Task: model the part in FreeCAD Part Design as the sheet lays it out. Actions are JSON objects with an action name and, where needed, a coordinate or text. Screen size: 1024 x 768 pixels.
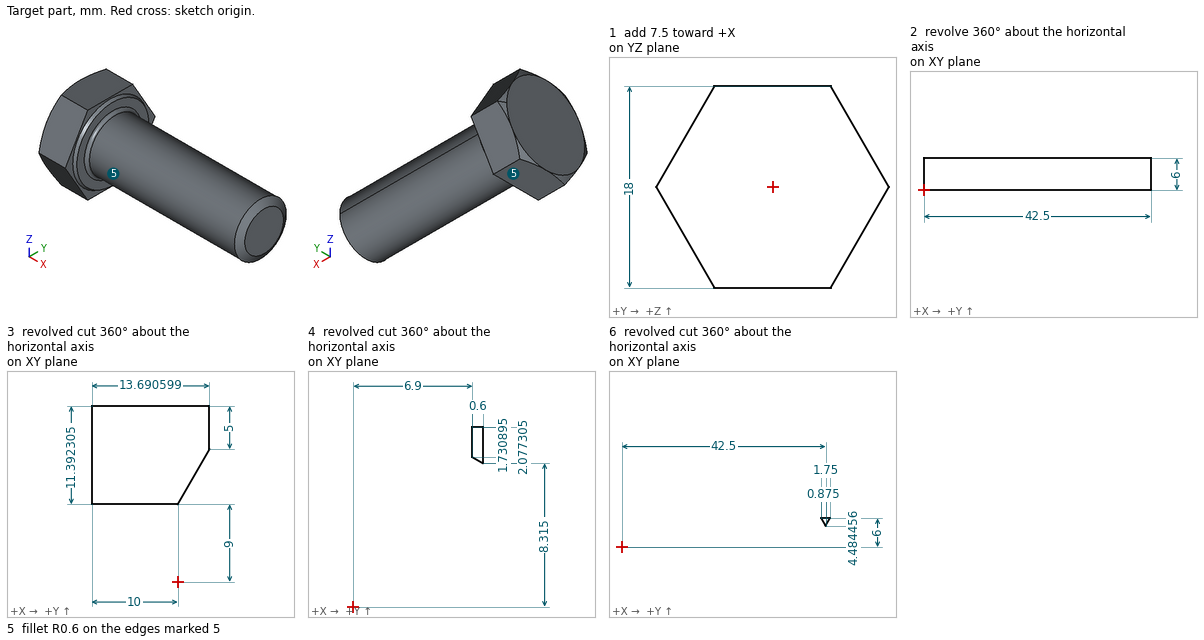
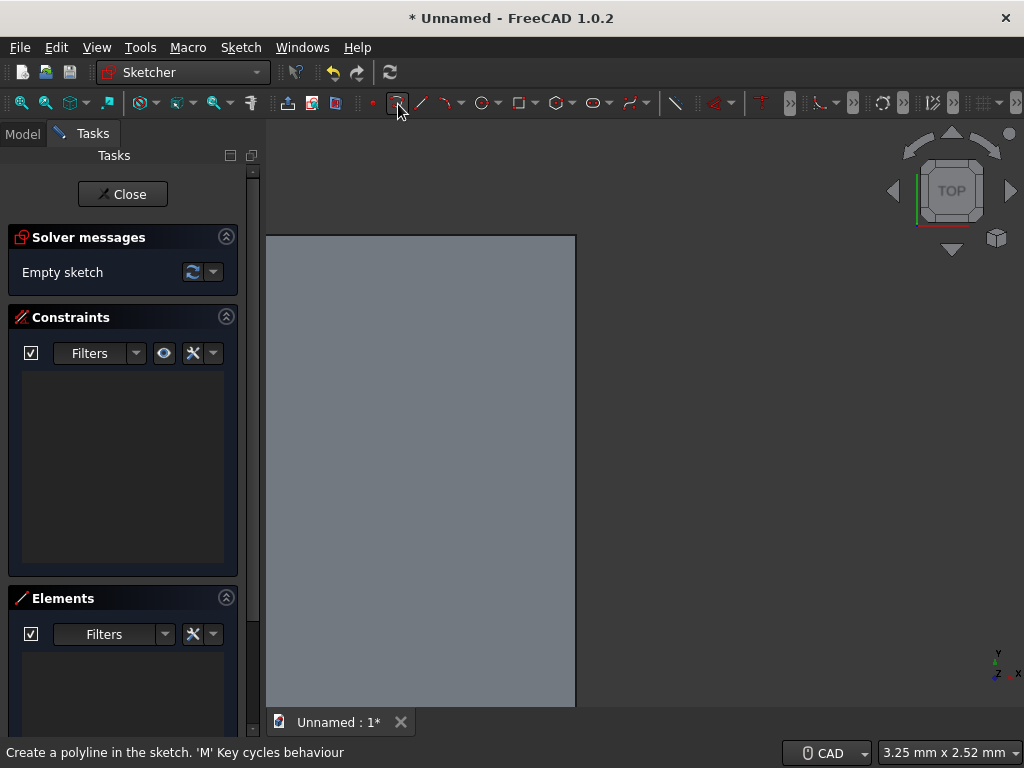
{"action": "left_click", "coordinate": [372, 235]}
{"action": "left_click", "coordinate": [576, 589]}
{"action": "left_click", "coordinate": [780, 235]}
{"action": "left_click", "coordinate": [372, 236]}
{"action": "key", "text": "Escape"}
{"action": "key", "text": "Escape"}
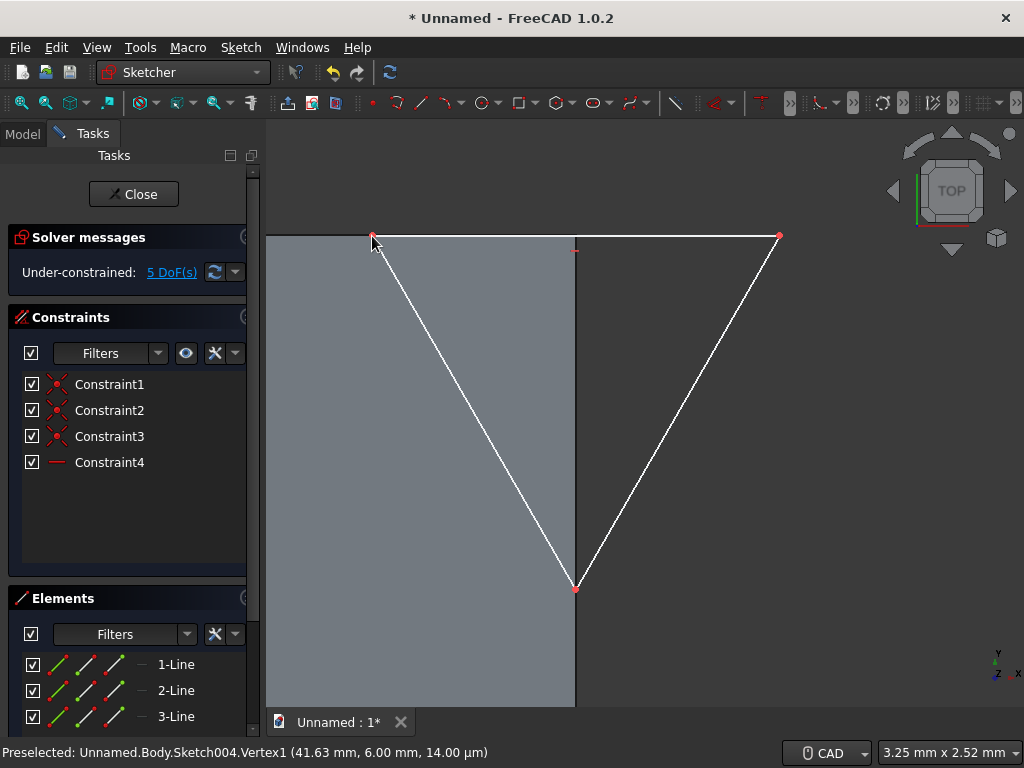
{"action": "left_click", "coordinate": [714, 104]}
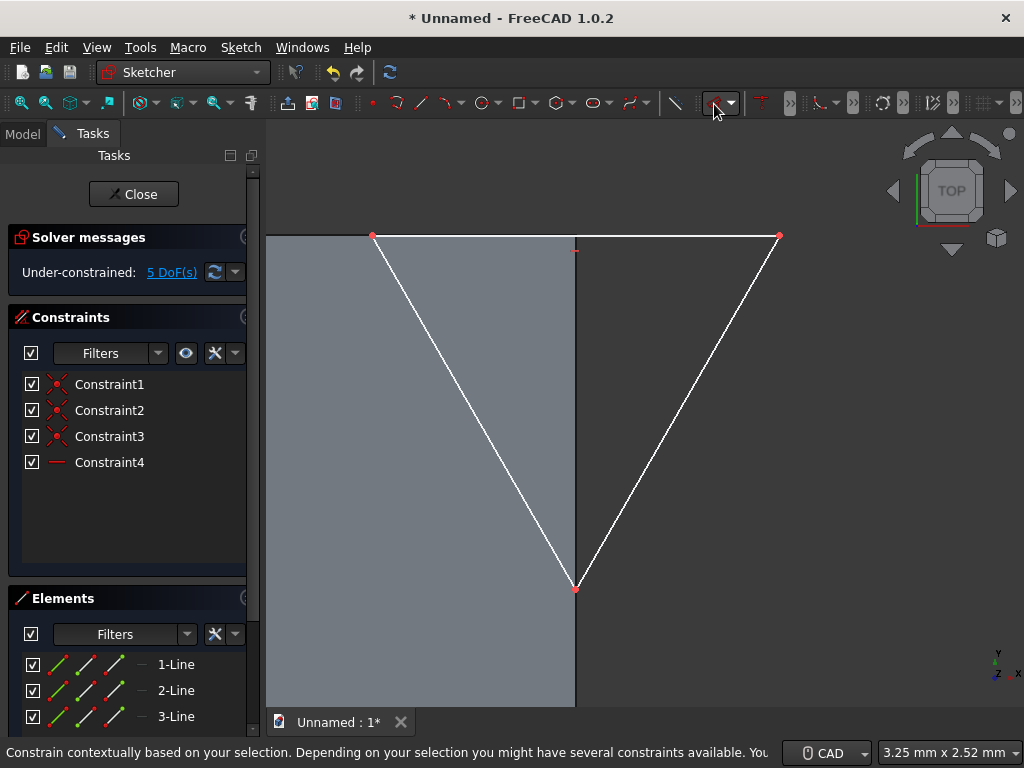
{"action": "left_click", "coordinate": [372, 236]}
{"action": "left_click", "coordinate": [406, 458]}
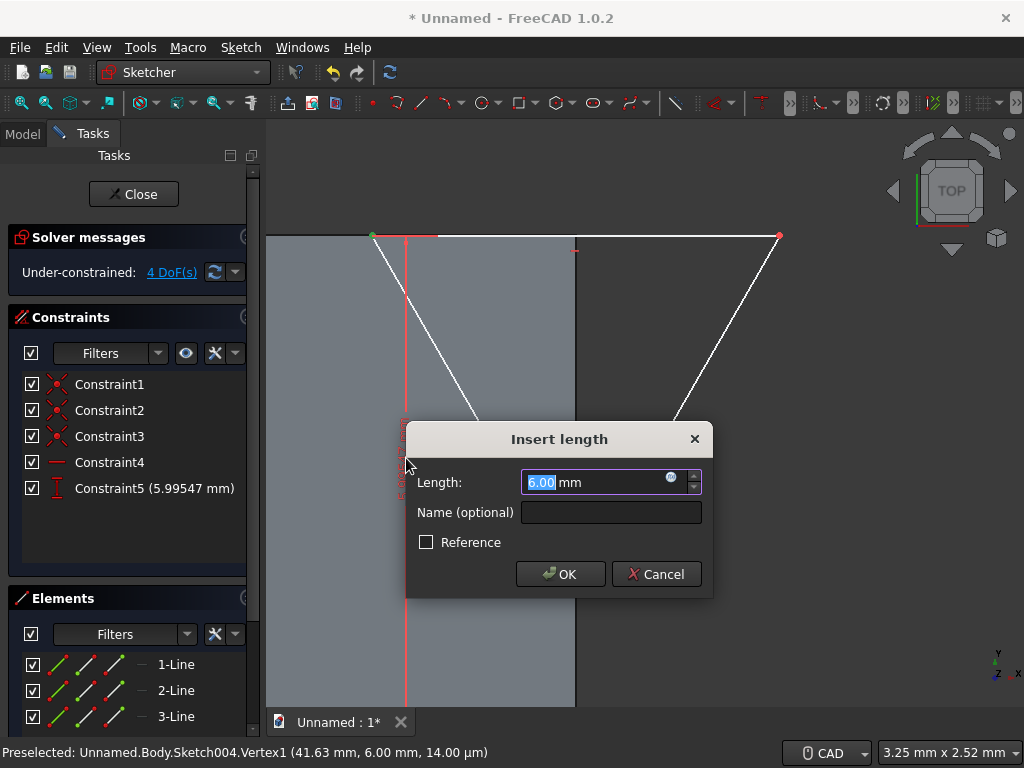
{"action": "type", "text": "6"}
{"action": "key", "text": "Return"}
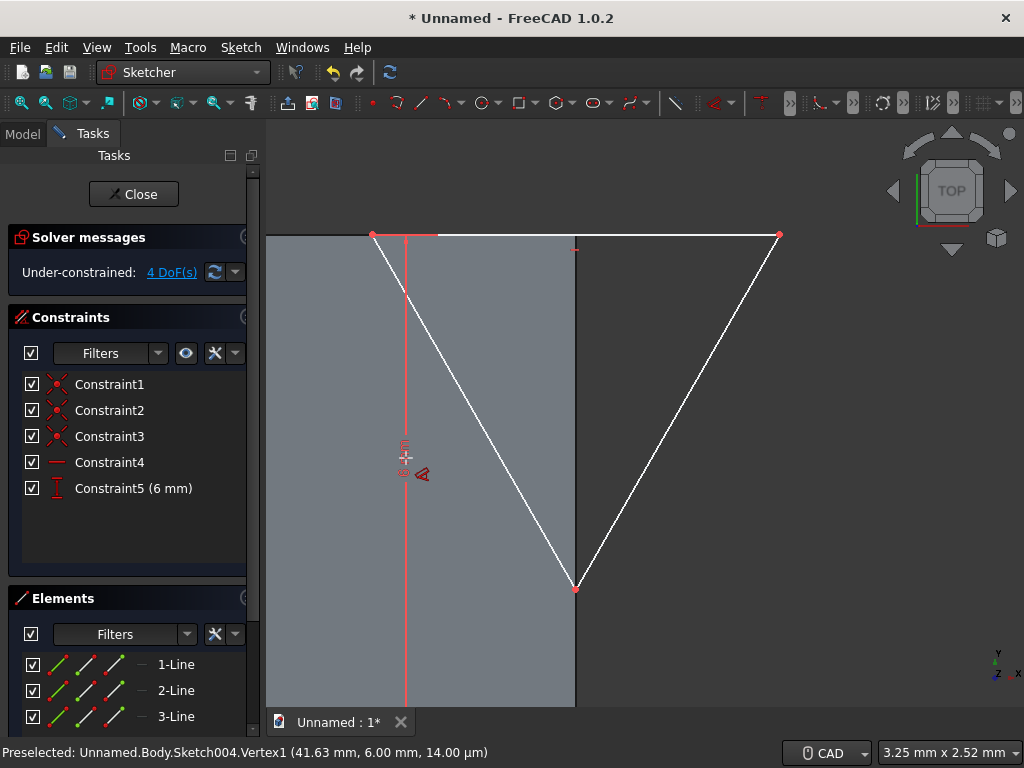
{"action": "left_click", "coordinate": [658, 235]}
{"action": "left_click", "coordinate": [576, 201]}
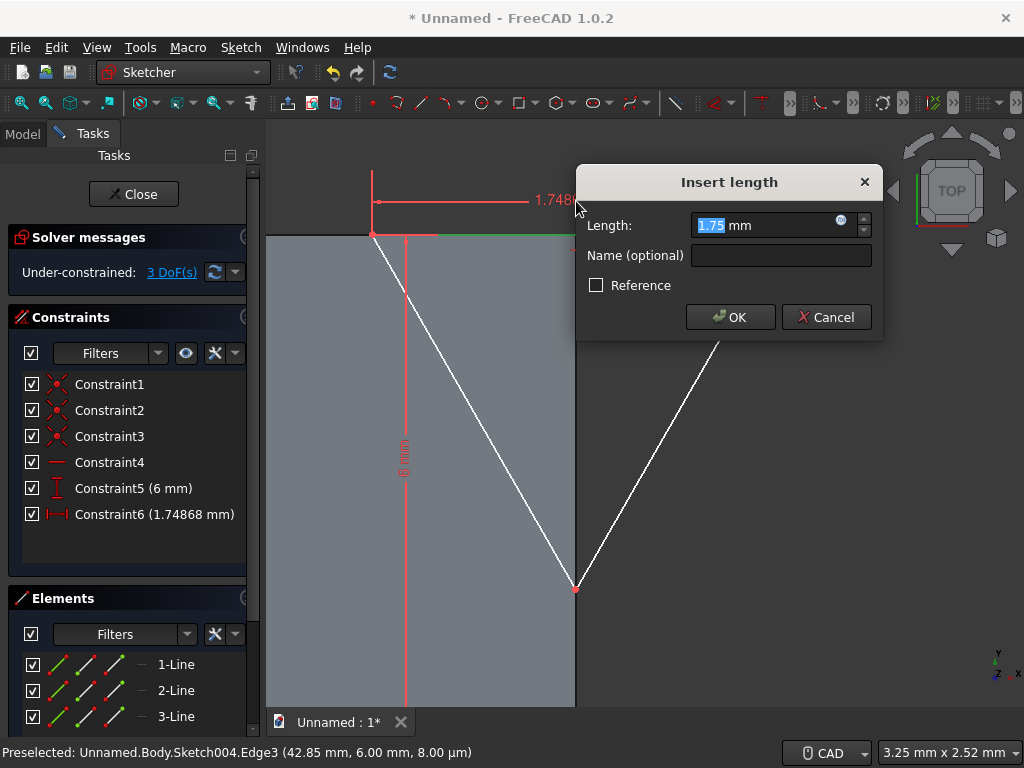
{"action": "type", "text": "1.75"}
{"action": "key", "text": "Return"}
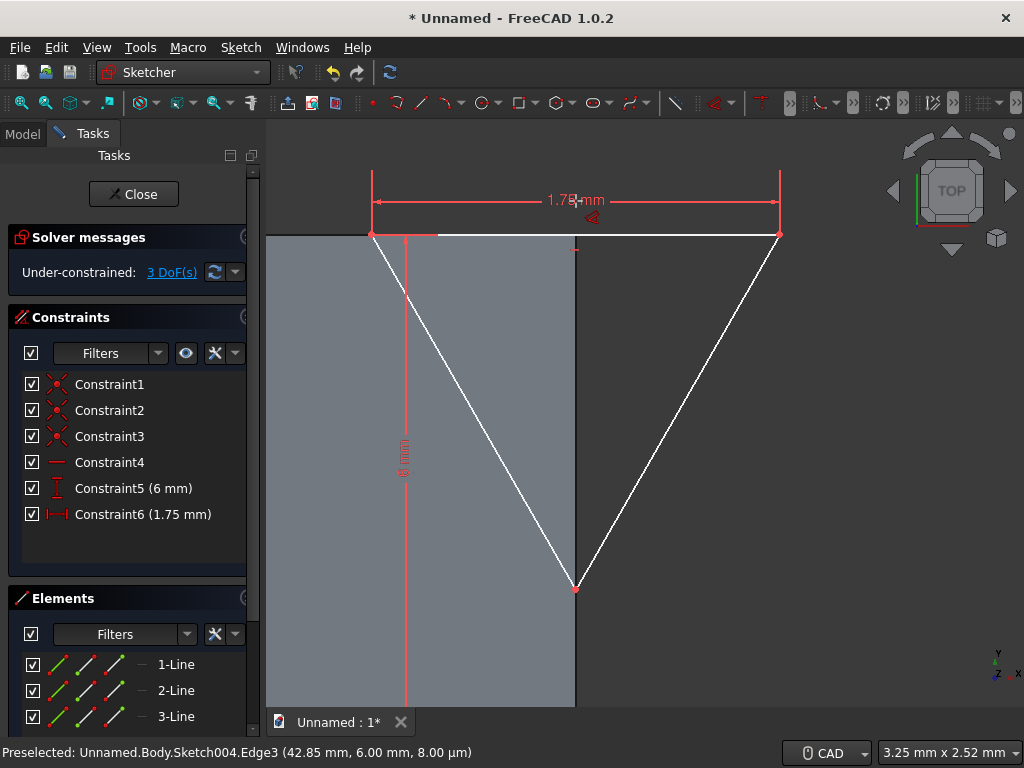
{"action": "left_click", "coordinate": [576, 590]}
{"action": "left_click", "coordinate": [435, 556]}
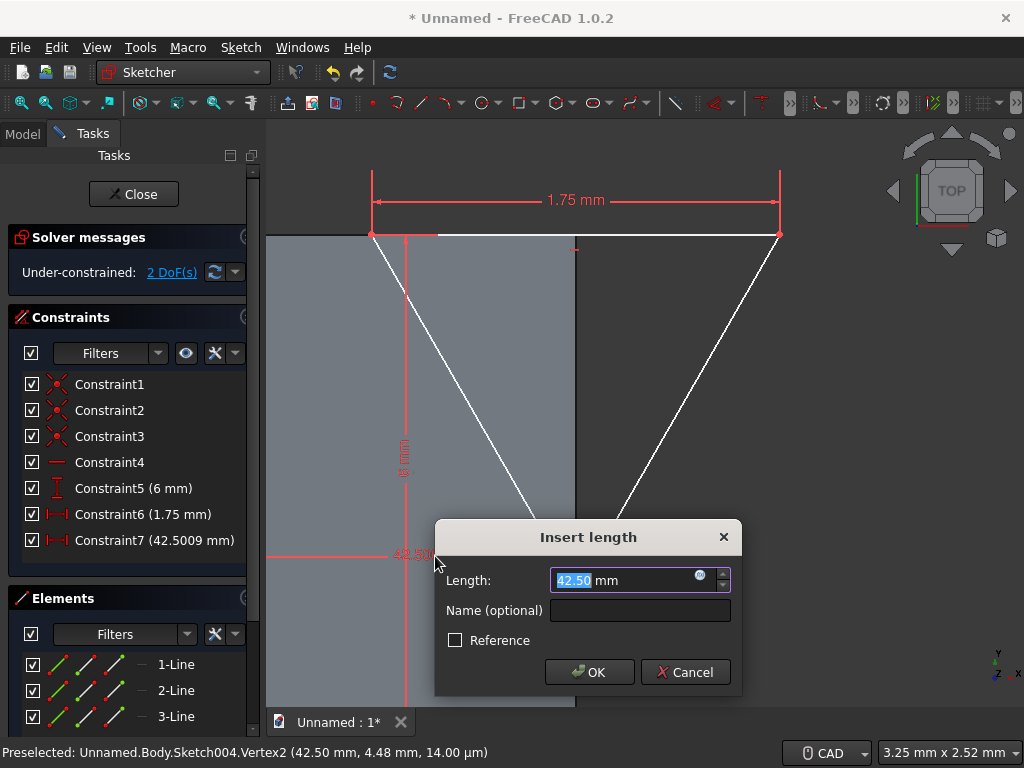
{"action": "type", "text": "42.5"}
{"action": "key", "text": "Return"}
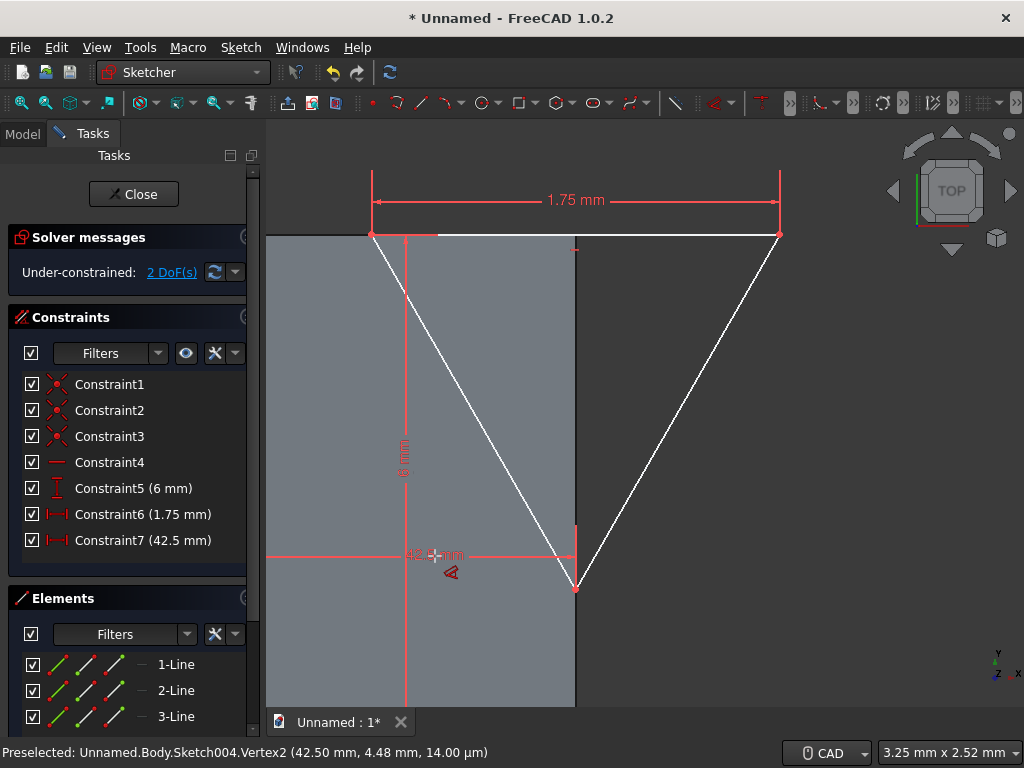
{"action": "left_click", "coordinate": [433, 341]}
{"action": "left_click", "coordinate": [474, 624]}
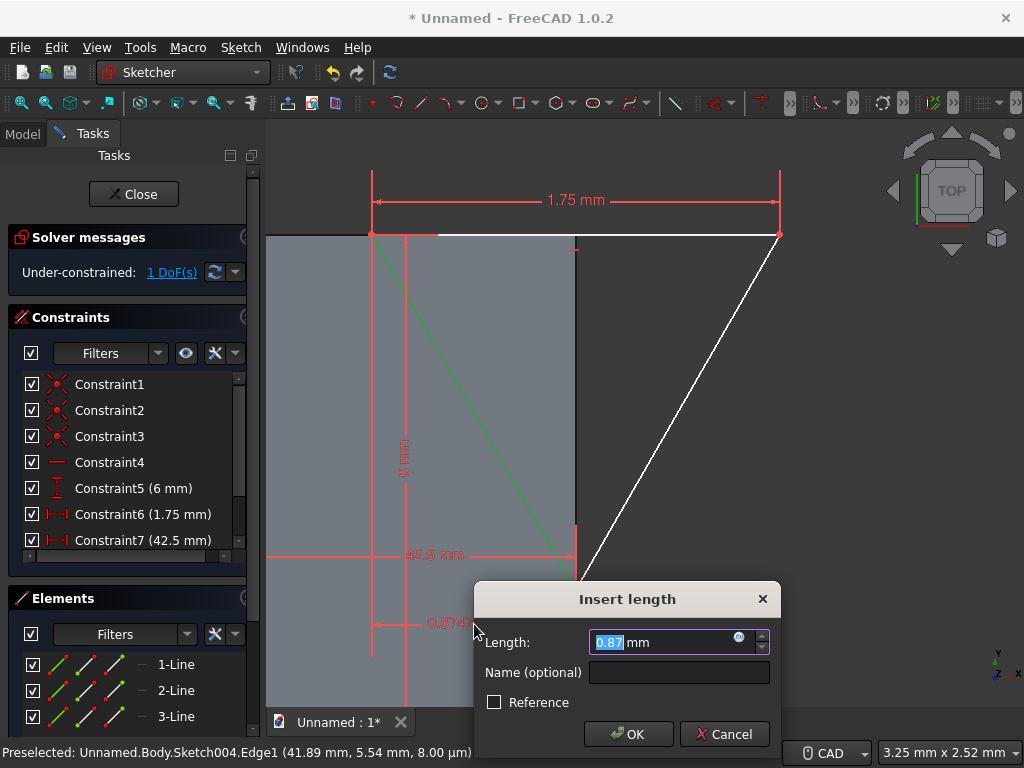
{"action": "type", "text": "0.875"}
{"action": "key", "text": "Return"}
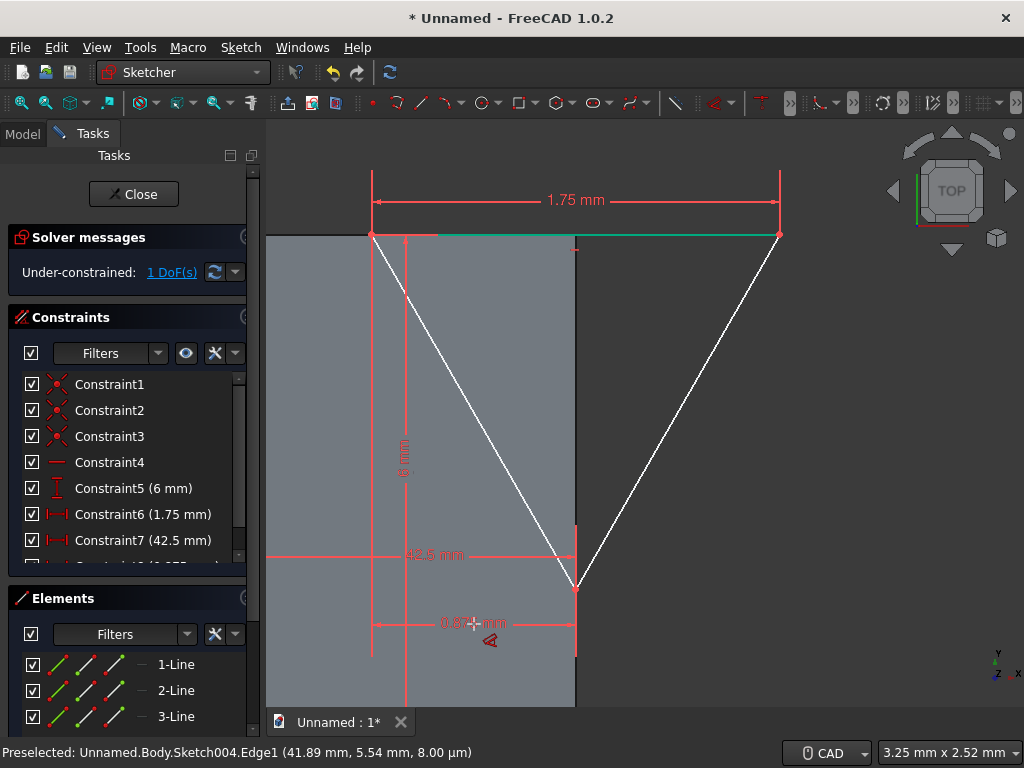
{"action": "left_click", "coordinate": [576, 590]}
{"action": "left_click", "coordinate": [610, 634]}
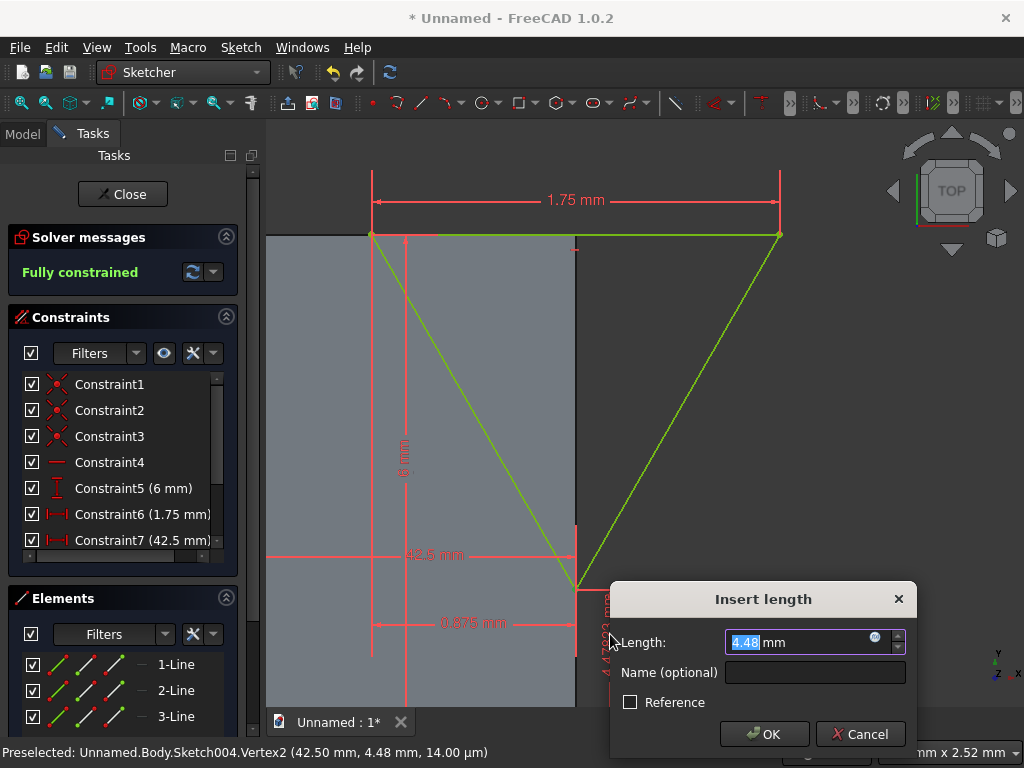
{"action": "type", "text": "4.484456"}
{"action": "key", "text": "Return"}
{"action": "key", "text": "Escape"}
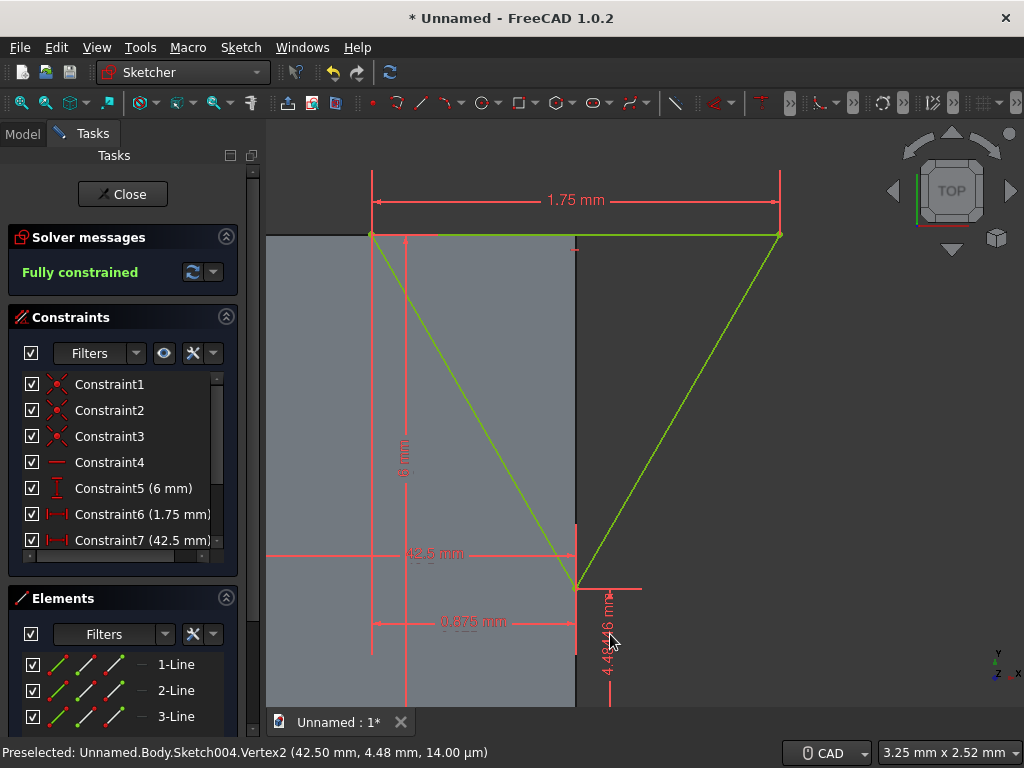
{"action": "left_click", "coordinate": [123, 194]}